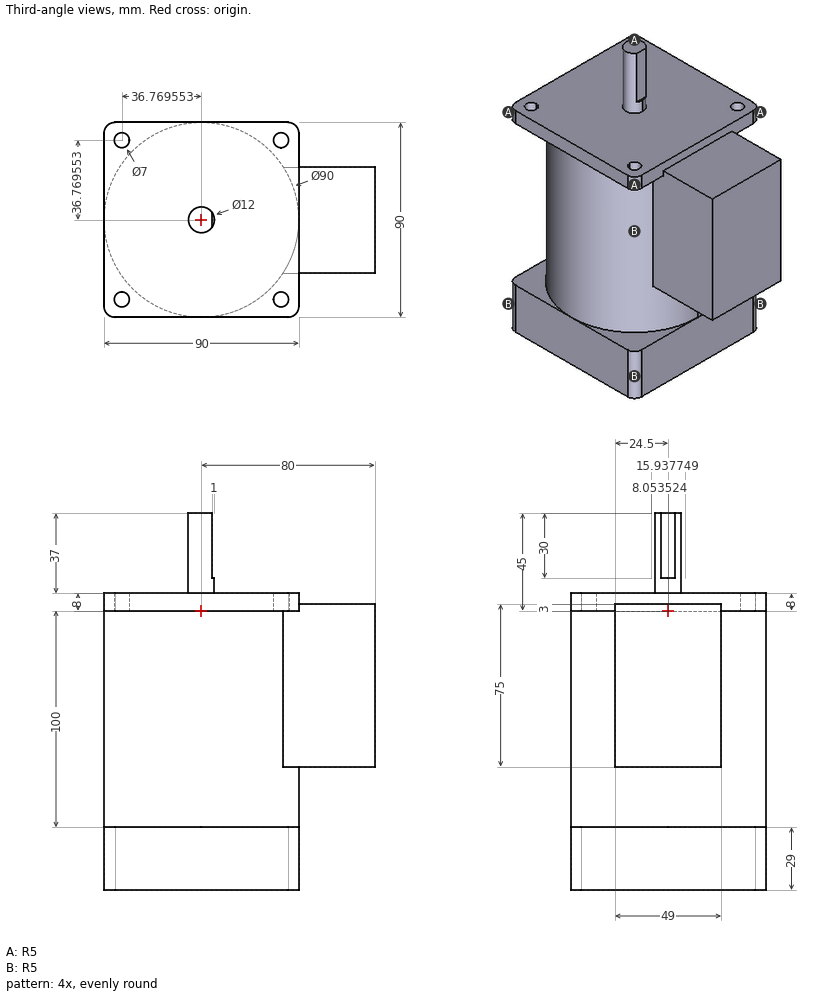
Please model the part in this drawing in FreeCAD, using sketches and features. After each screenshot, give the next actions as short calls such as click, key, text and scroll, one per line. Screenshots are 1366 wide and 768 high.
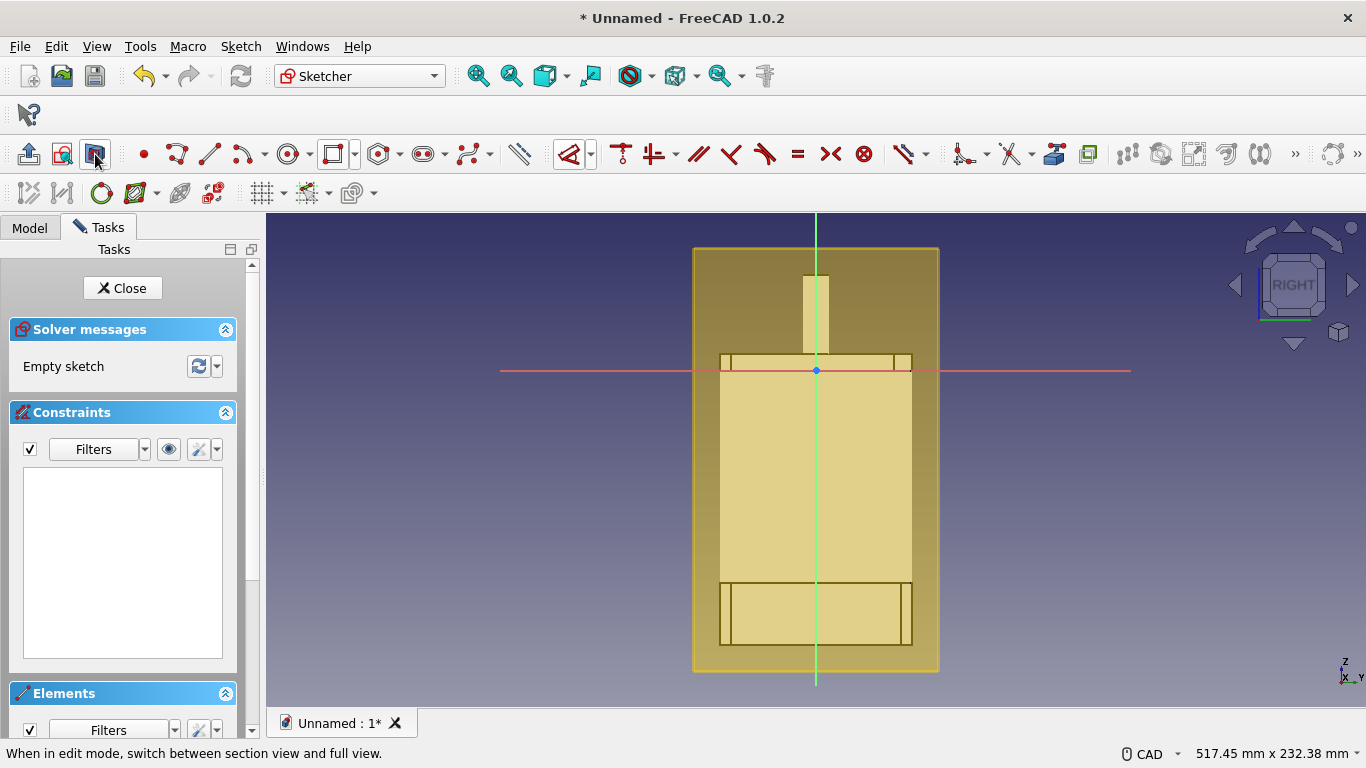
scroll(845, 264, up, 6)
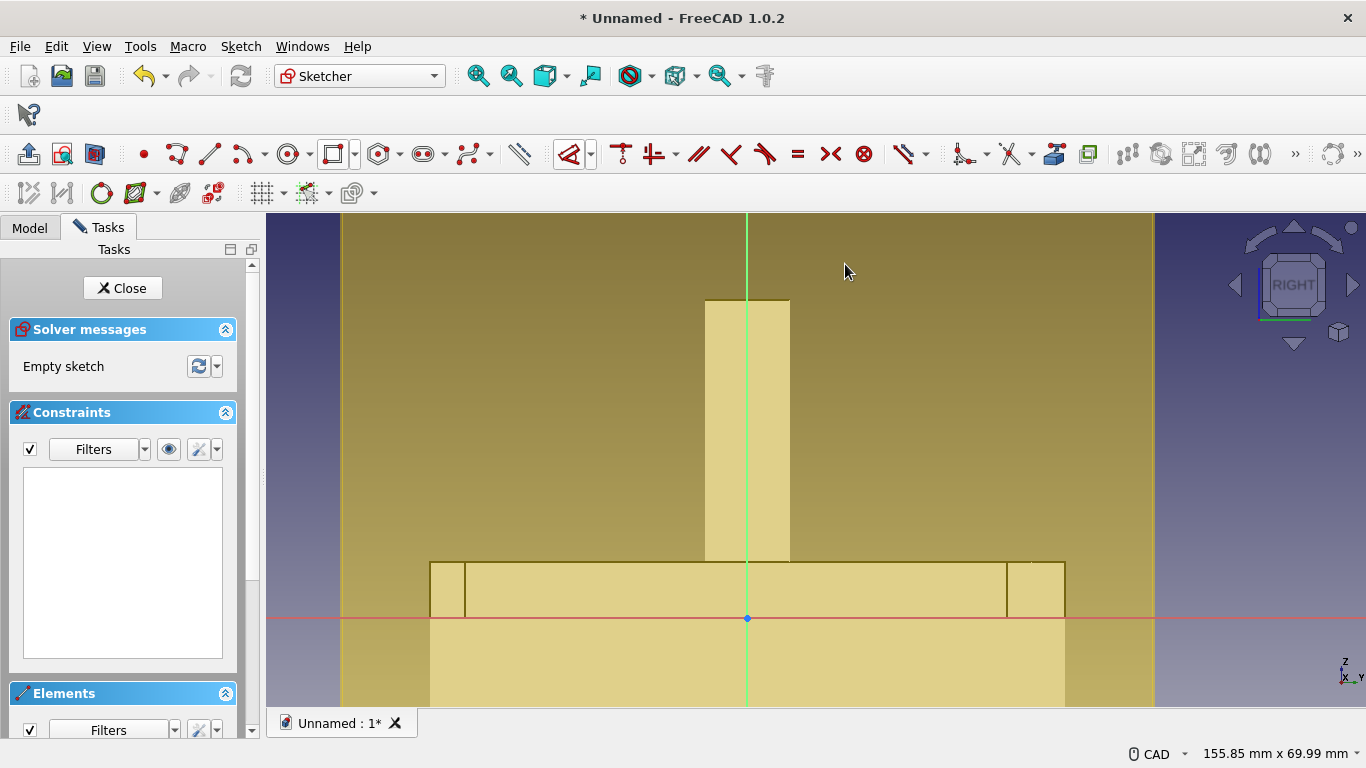
click(332, 154)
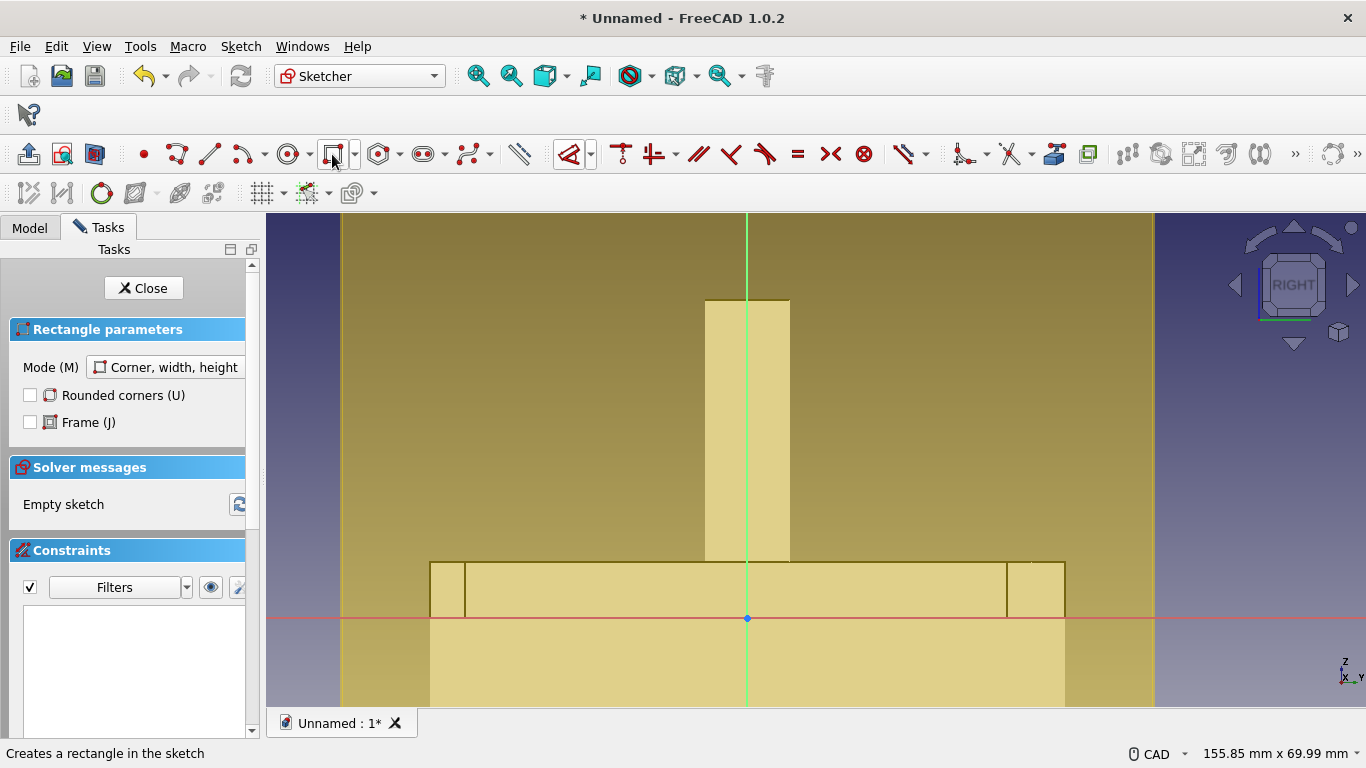
click(691, 300)
click(803, 512)
key(Escape)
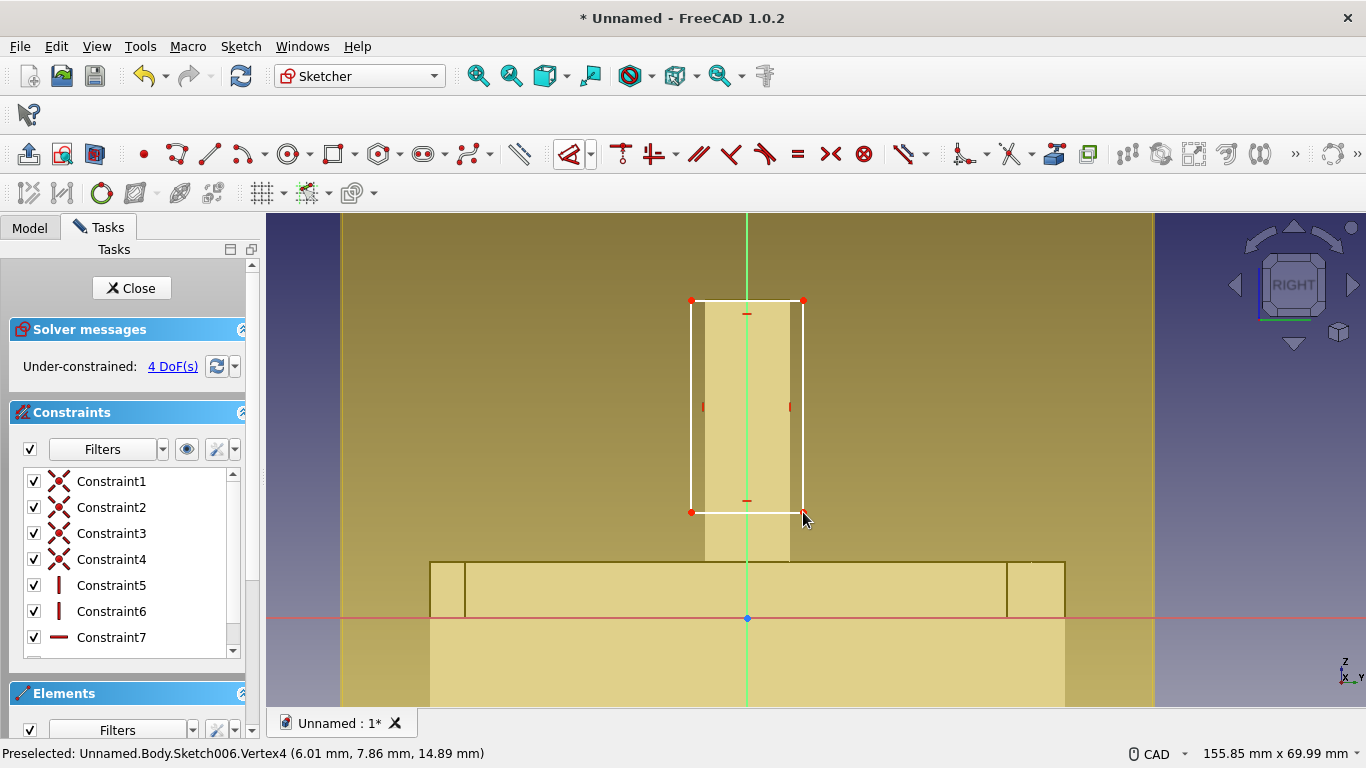
click(691, 365)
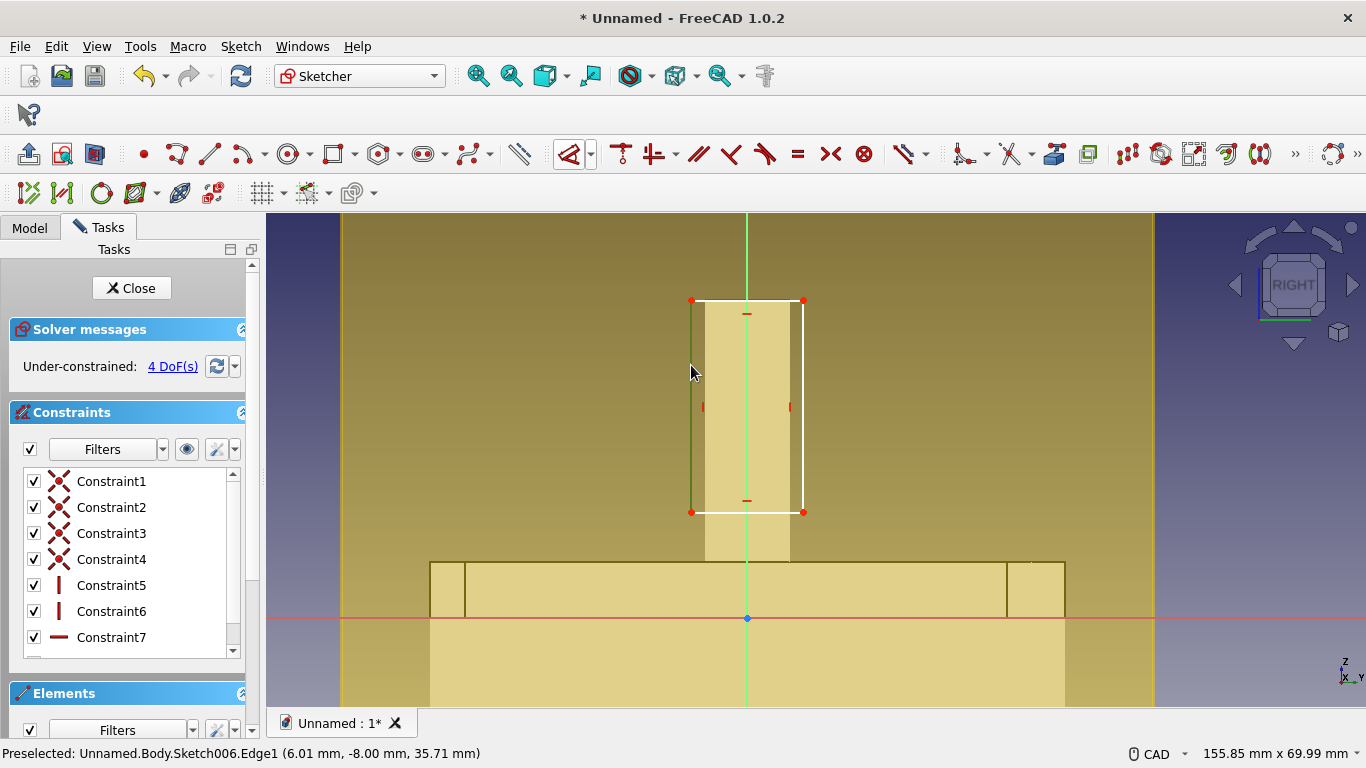
key(i)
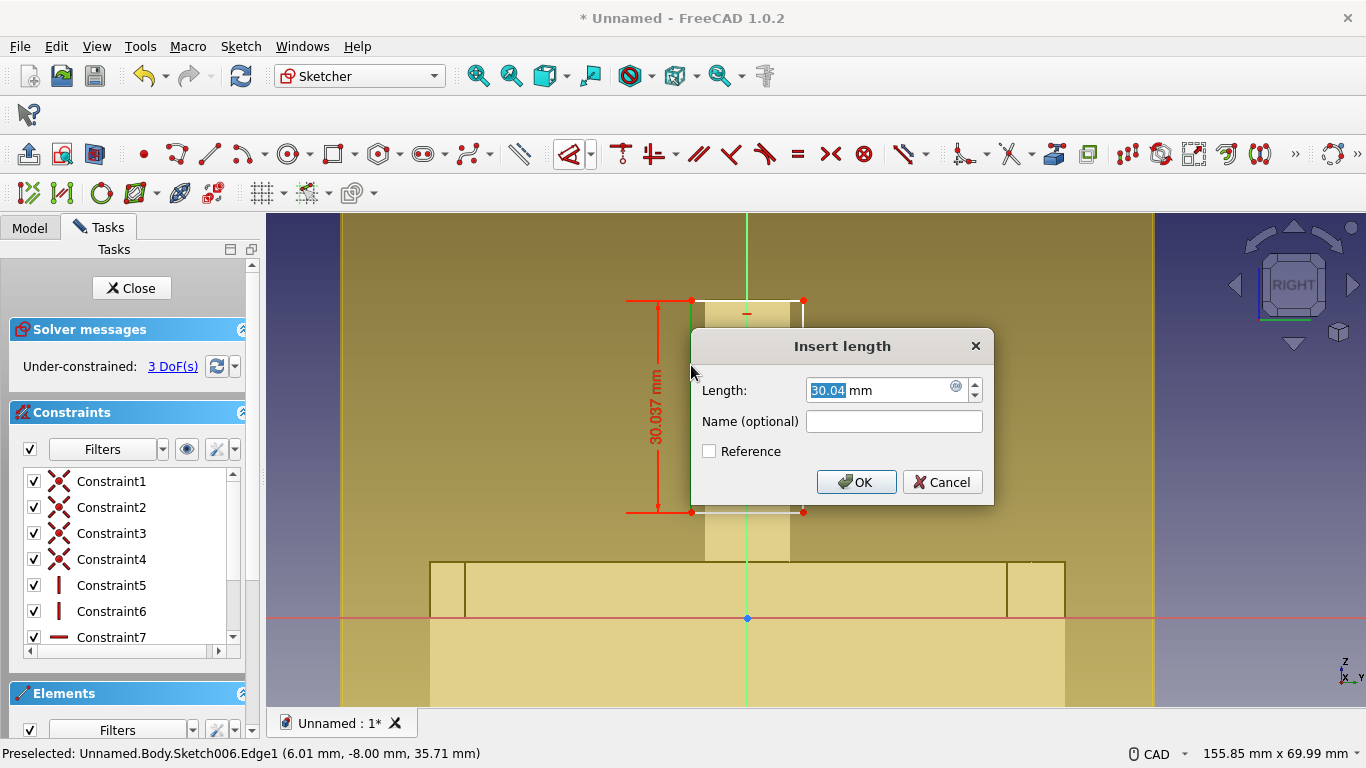
text(30)
key(Return)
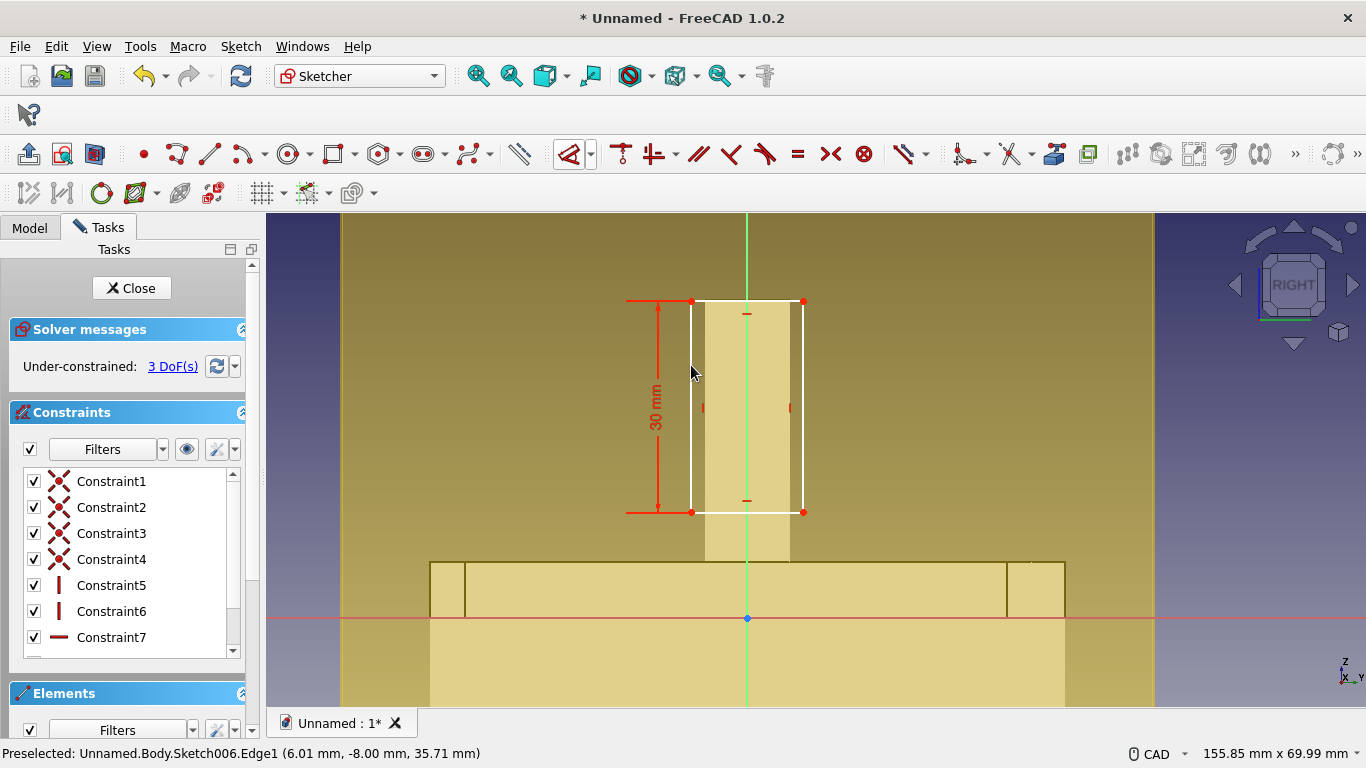
click(691, 301)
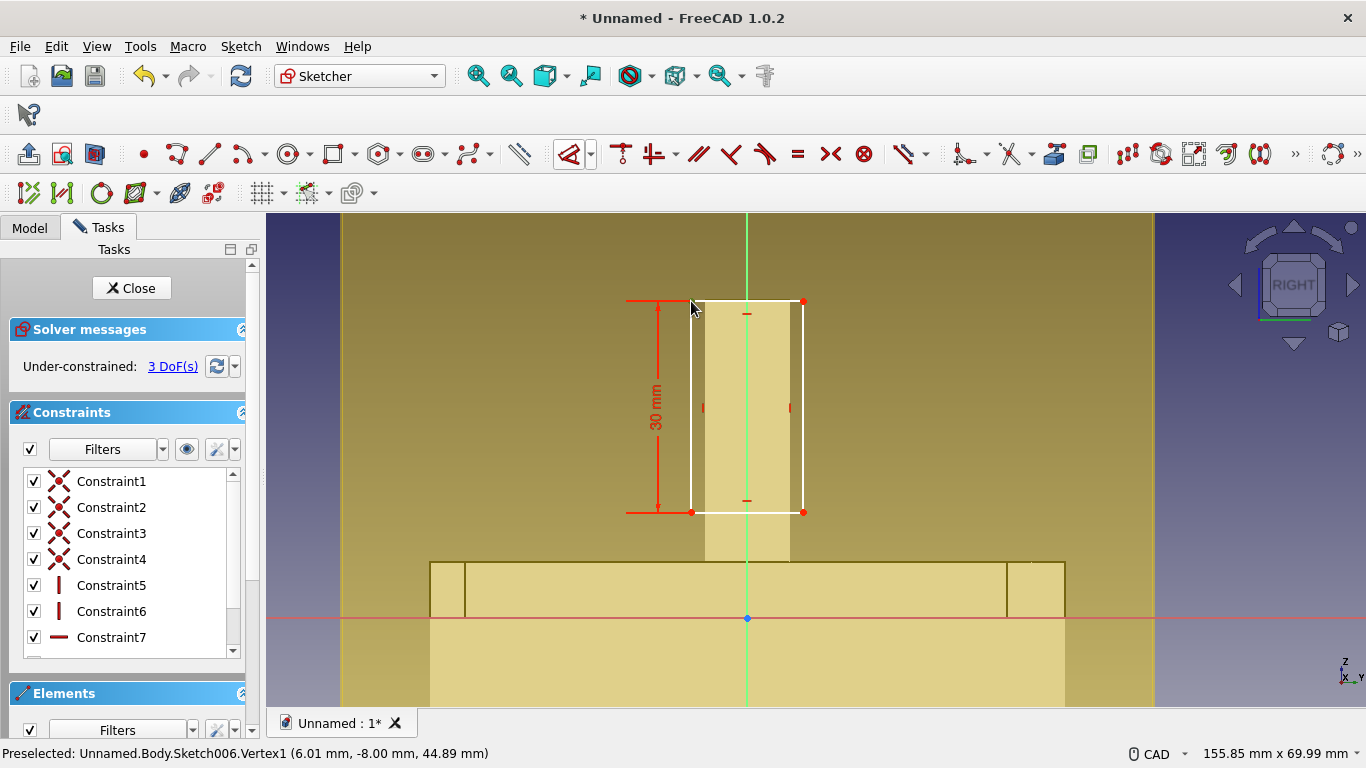
key(i)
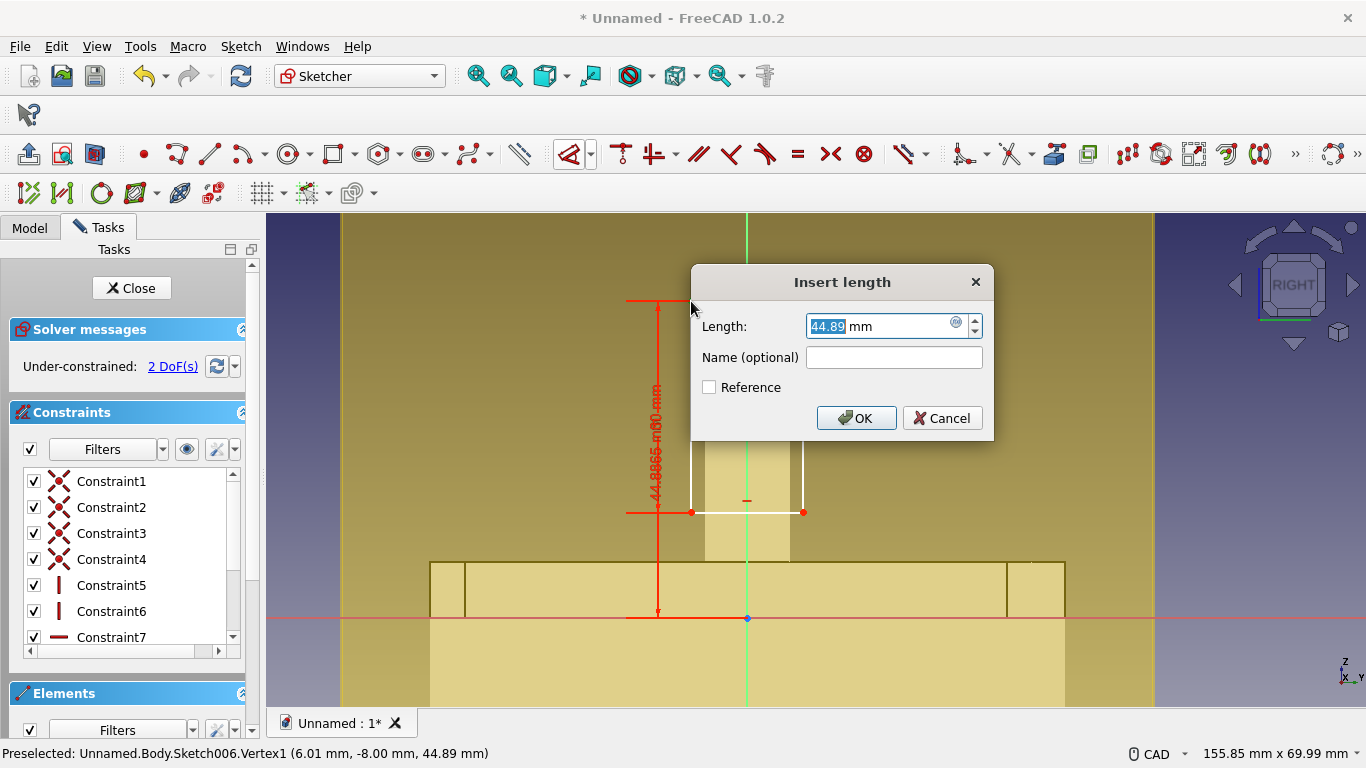
text(45)
key(Return)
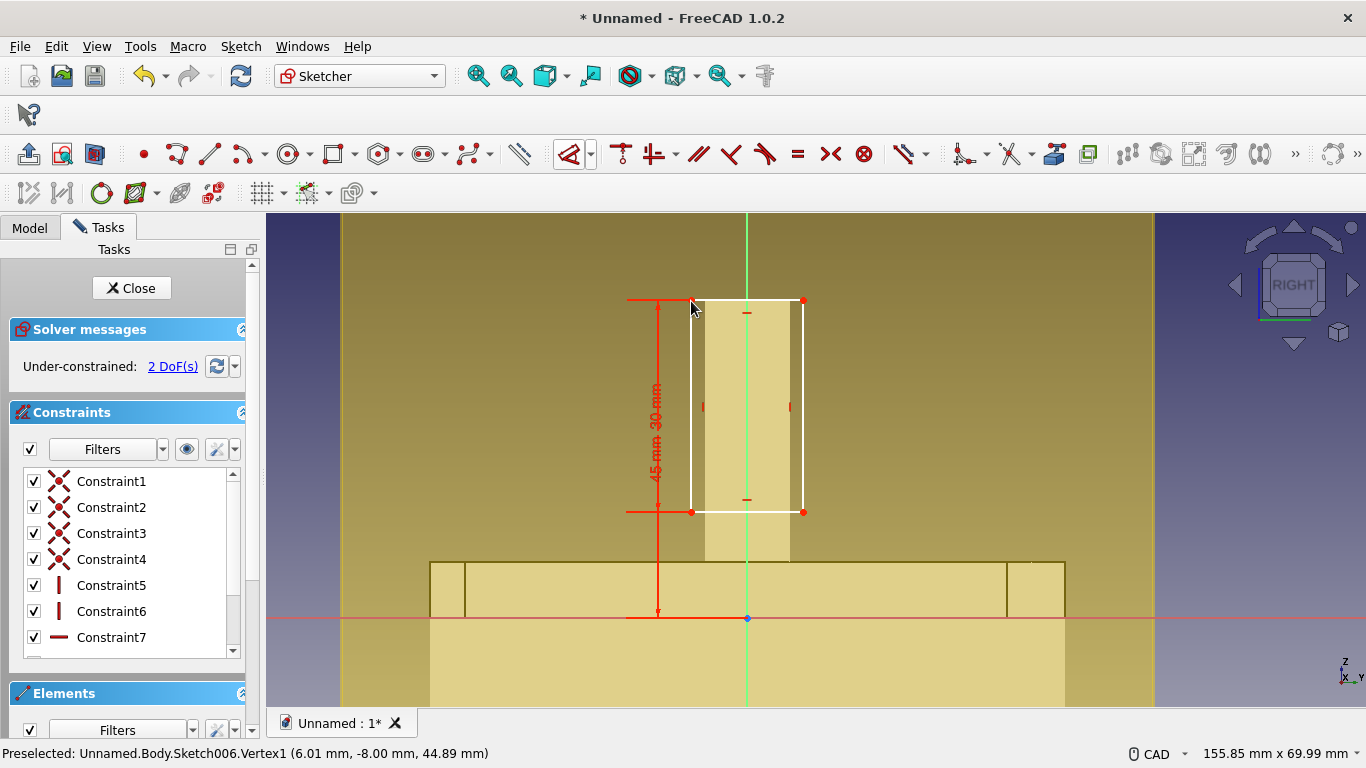
click(725, 512)